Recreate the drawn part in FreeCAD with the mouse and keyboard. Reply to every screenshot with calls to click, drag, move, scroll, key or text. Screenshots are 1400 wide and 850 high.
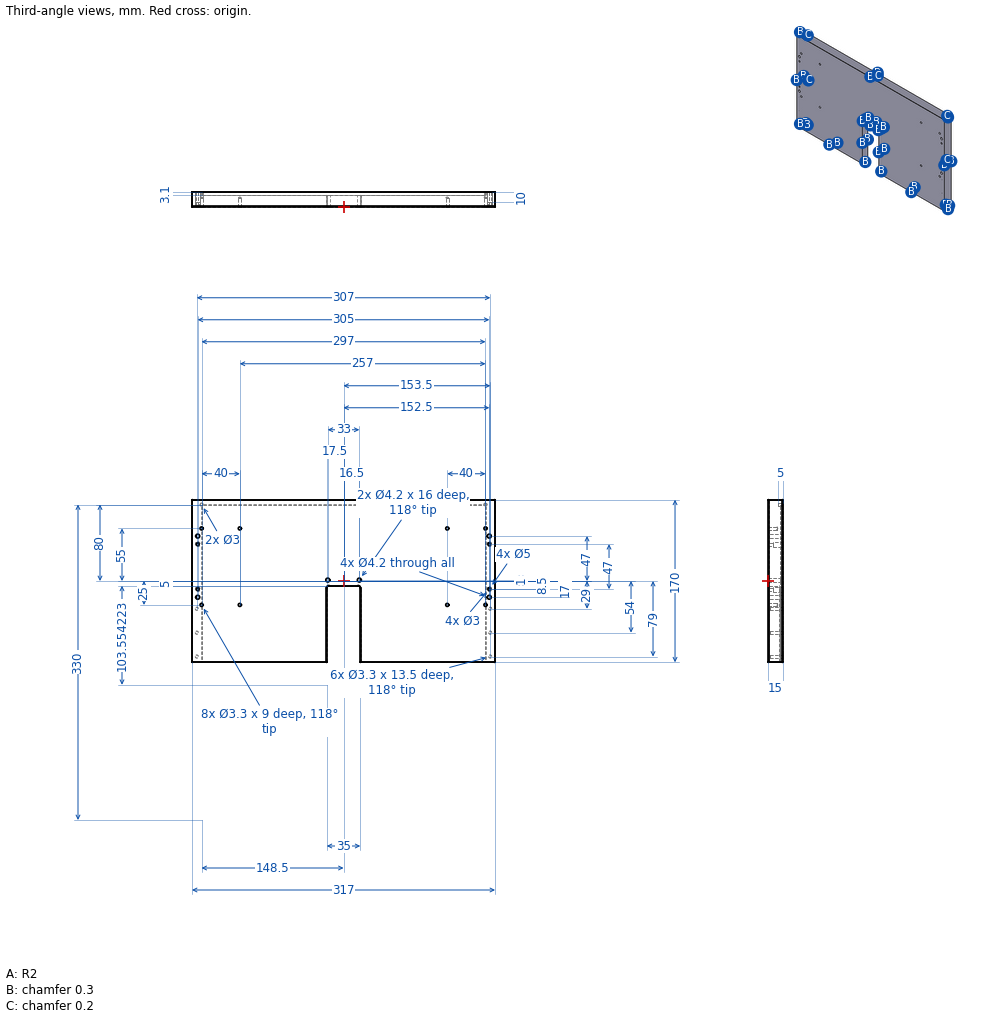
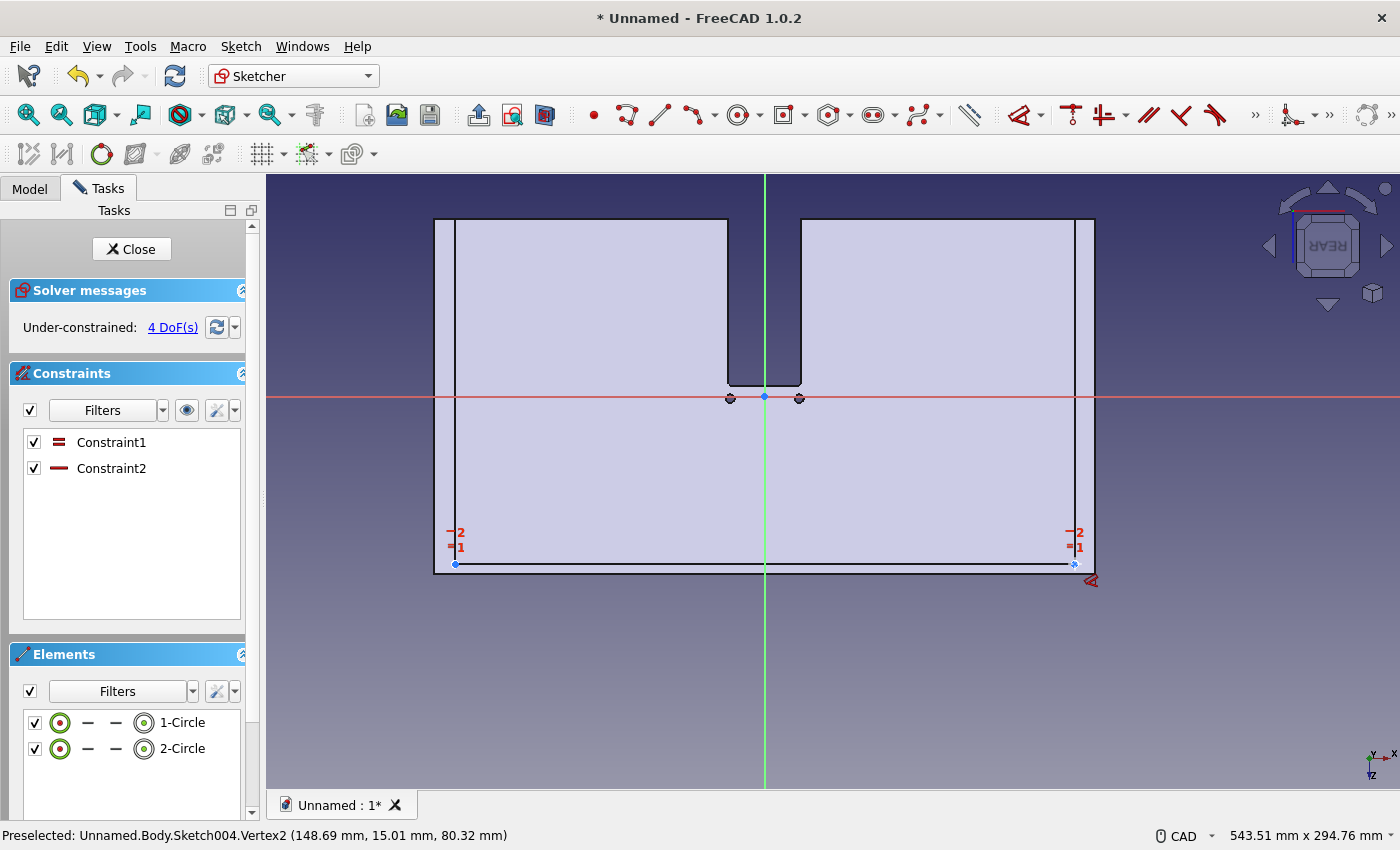
scroll(453, 562, up, 10)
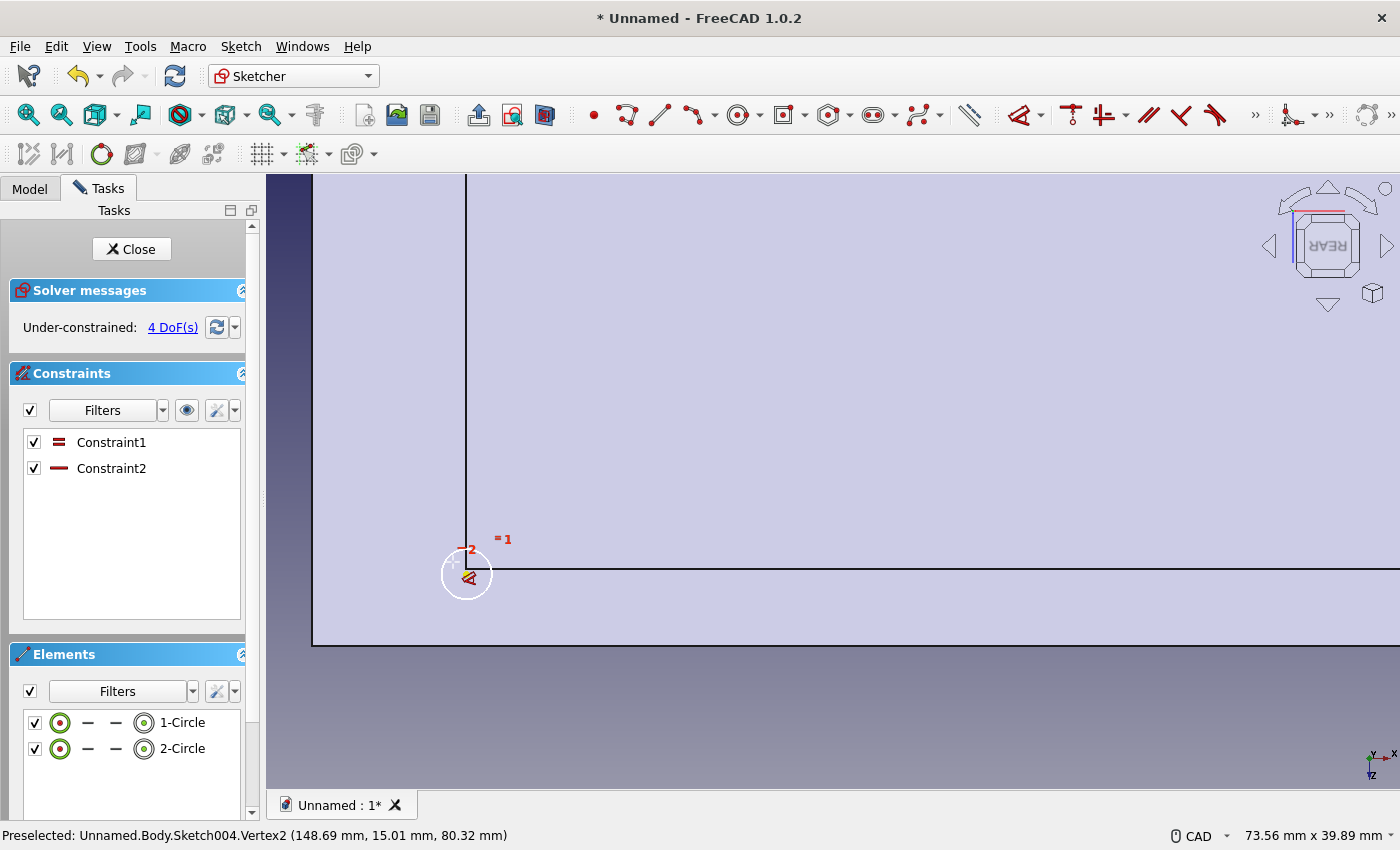
click(449, 557)
click(426, 535)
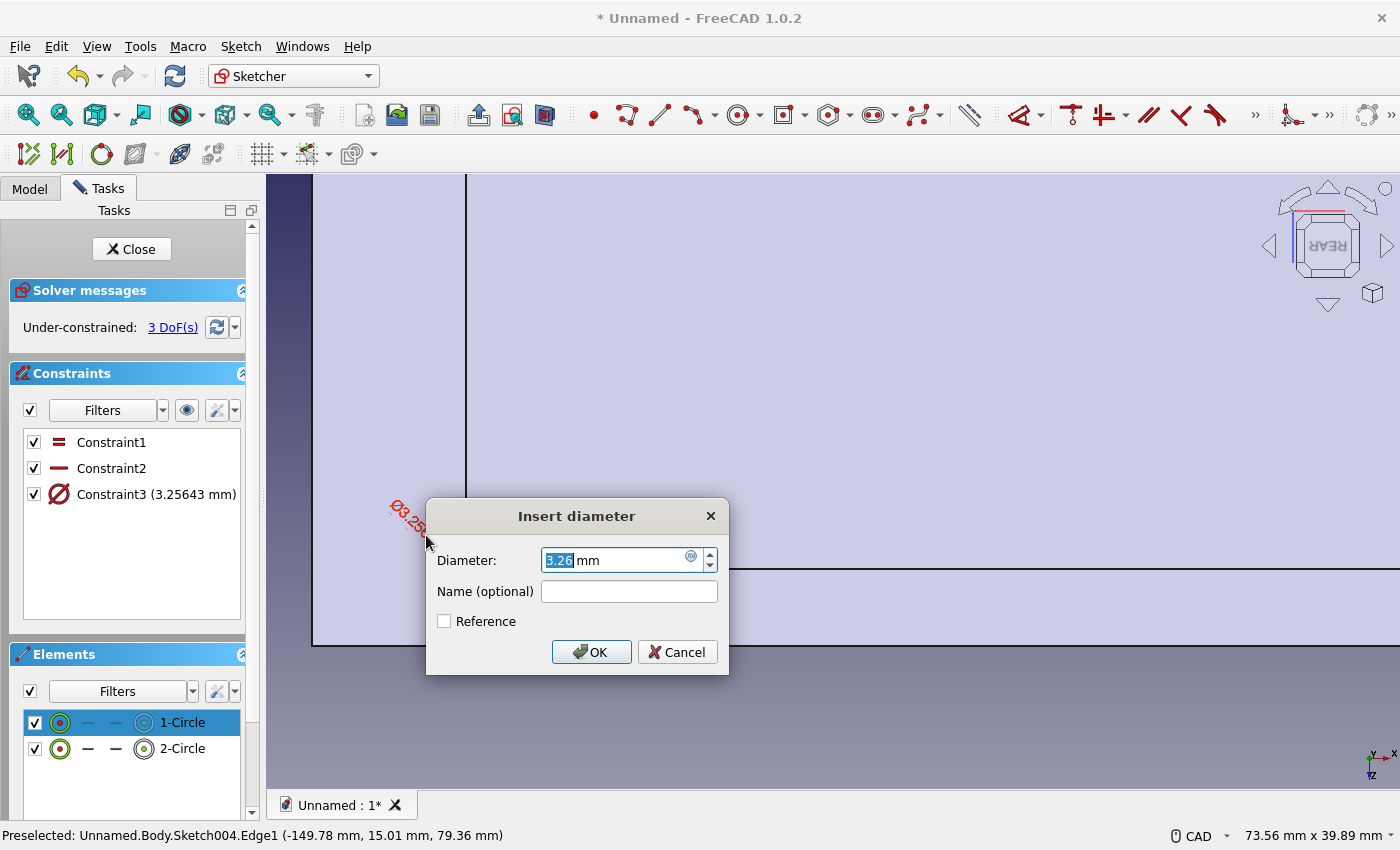
text(3)
key(Return)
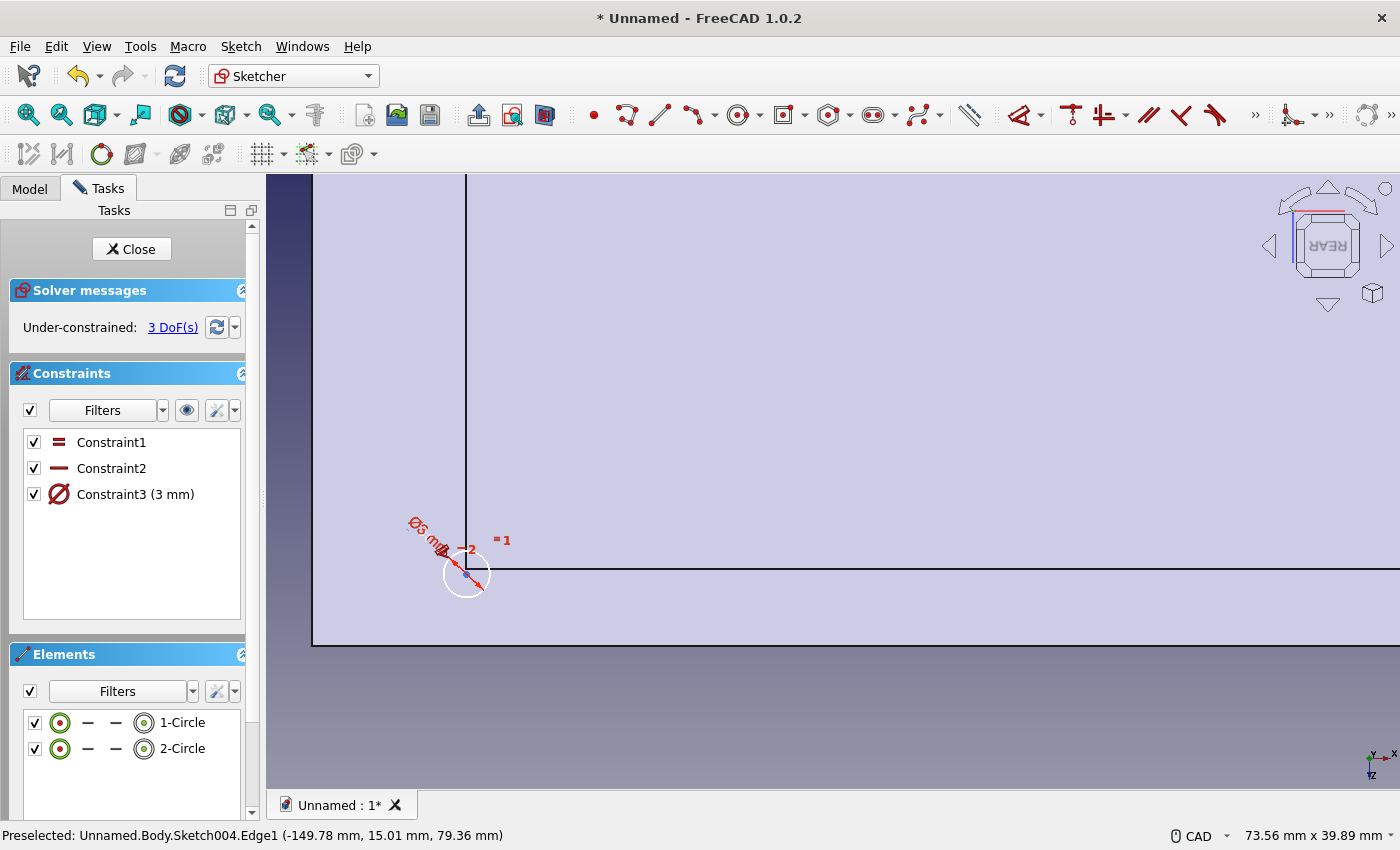
scroll(453, 562, down, 10)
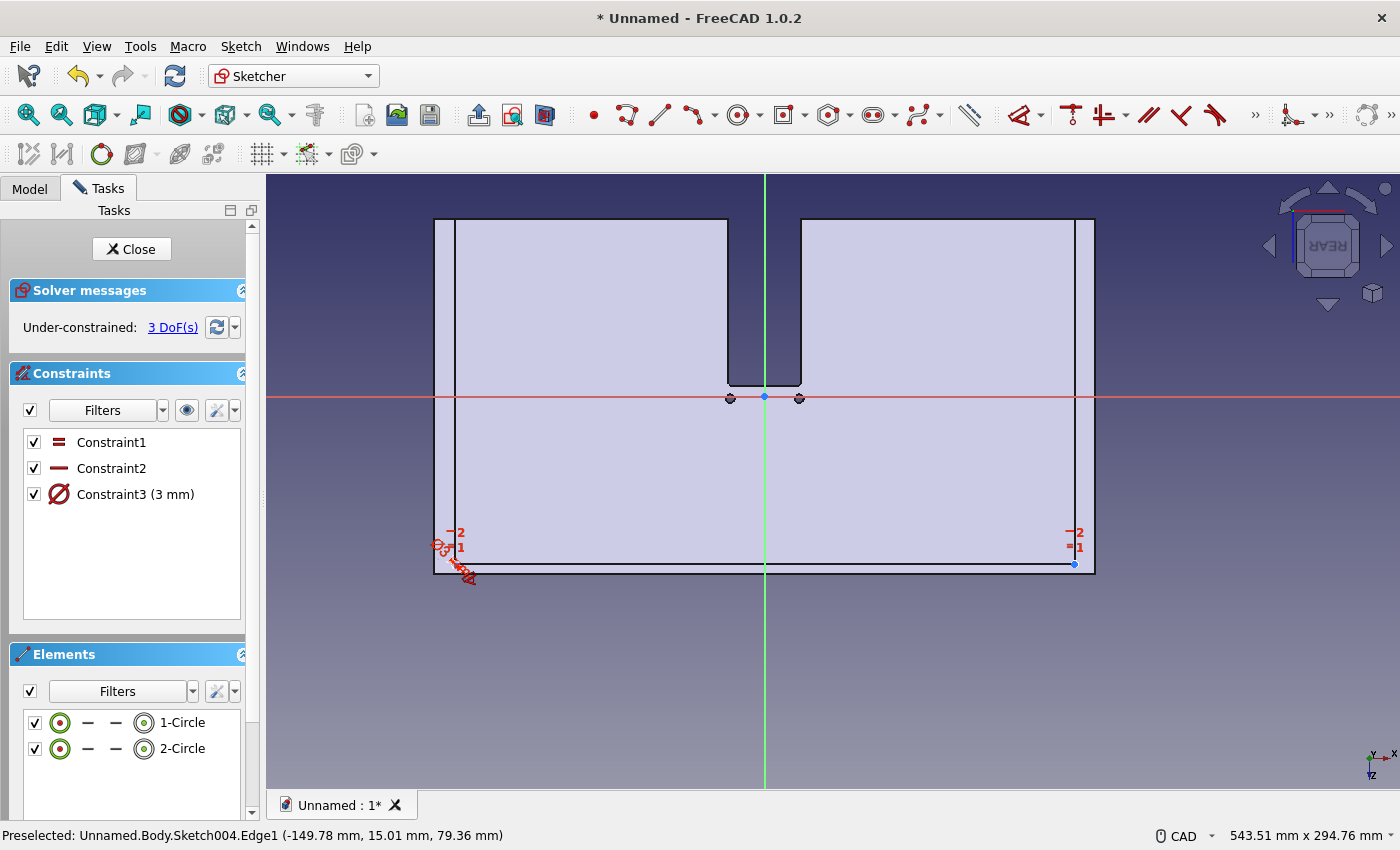
click(455, 564)
click(421, 480)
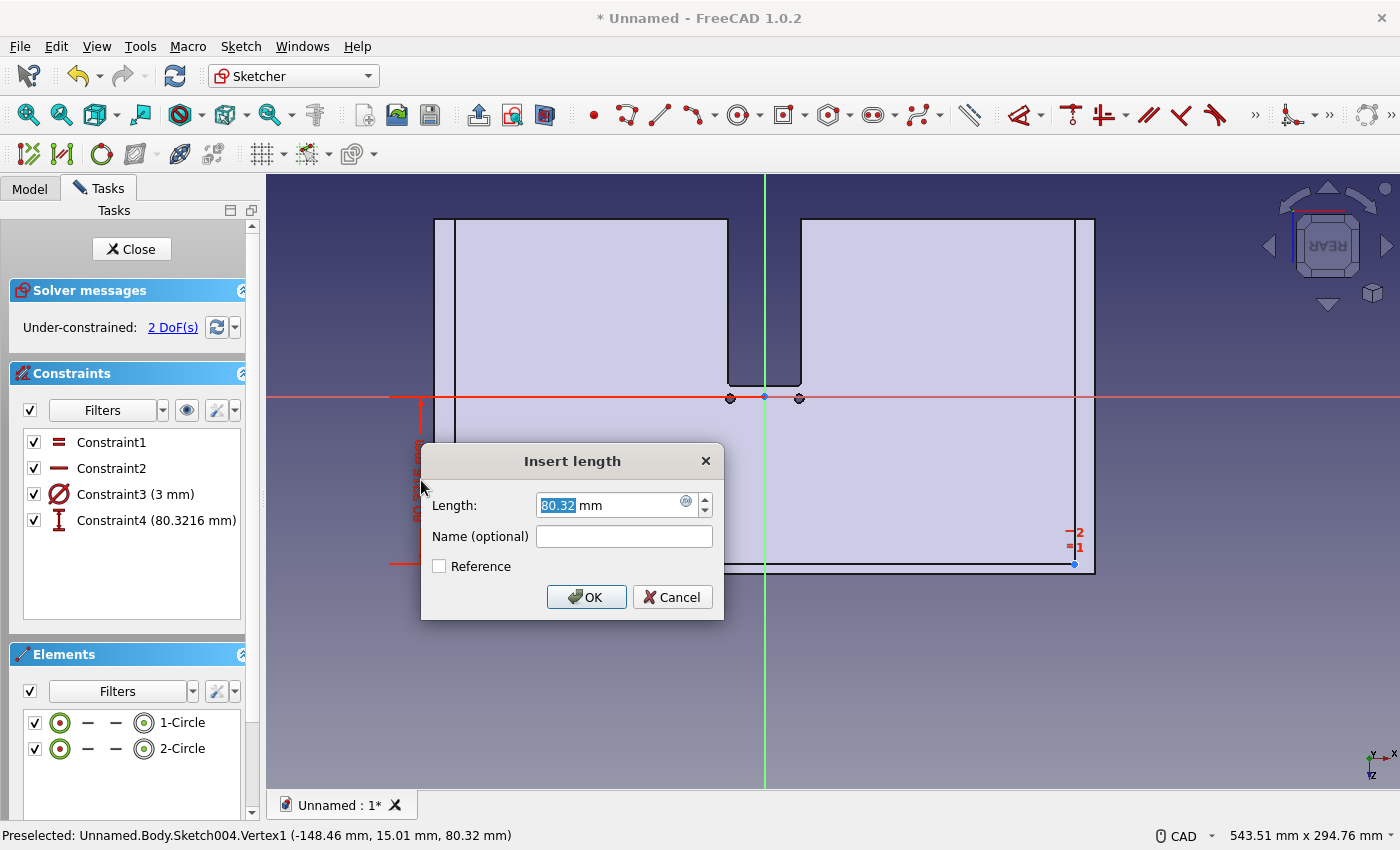
text(80)
key(Return)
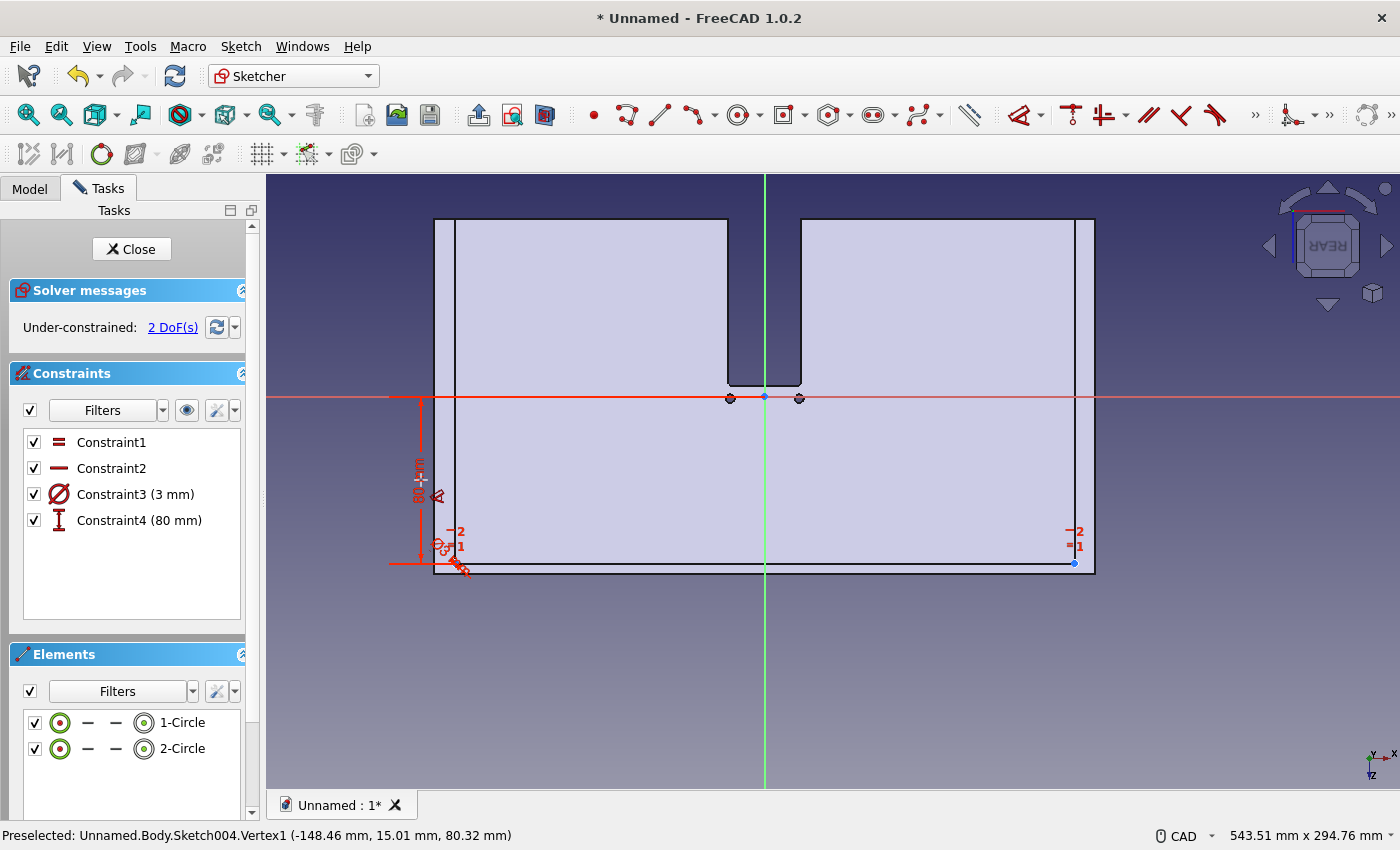
click(455, 564)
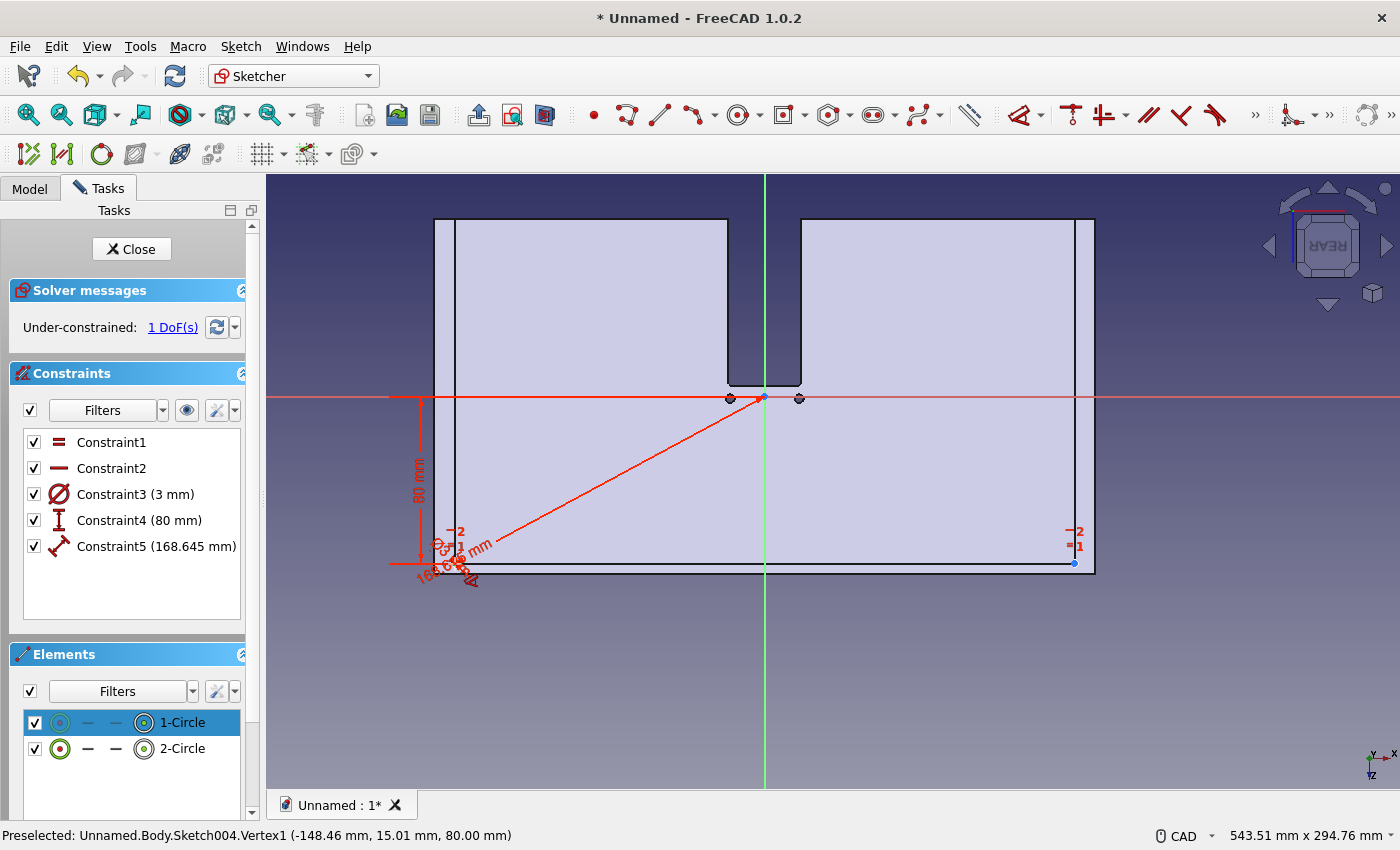
click(1075, 564)
click(622, 598)